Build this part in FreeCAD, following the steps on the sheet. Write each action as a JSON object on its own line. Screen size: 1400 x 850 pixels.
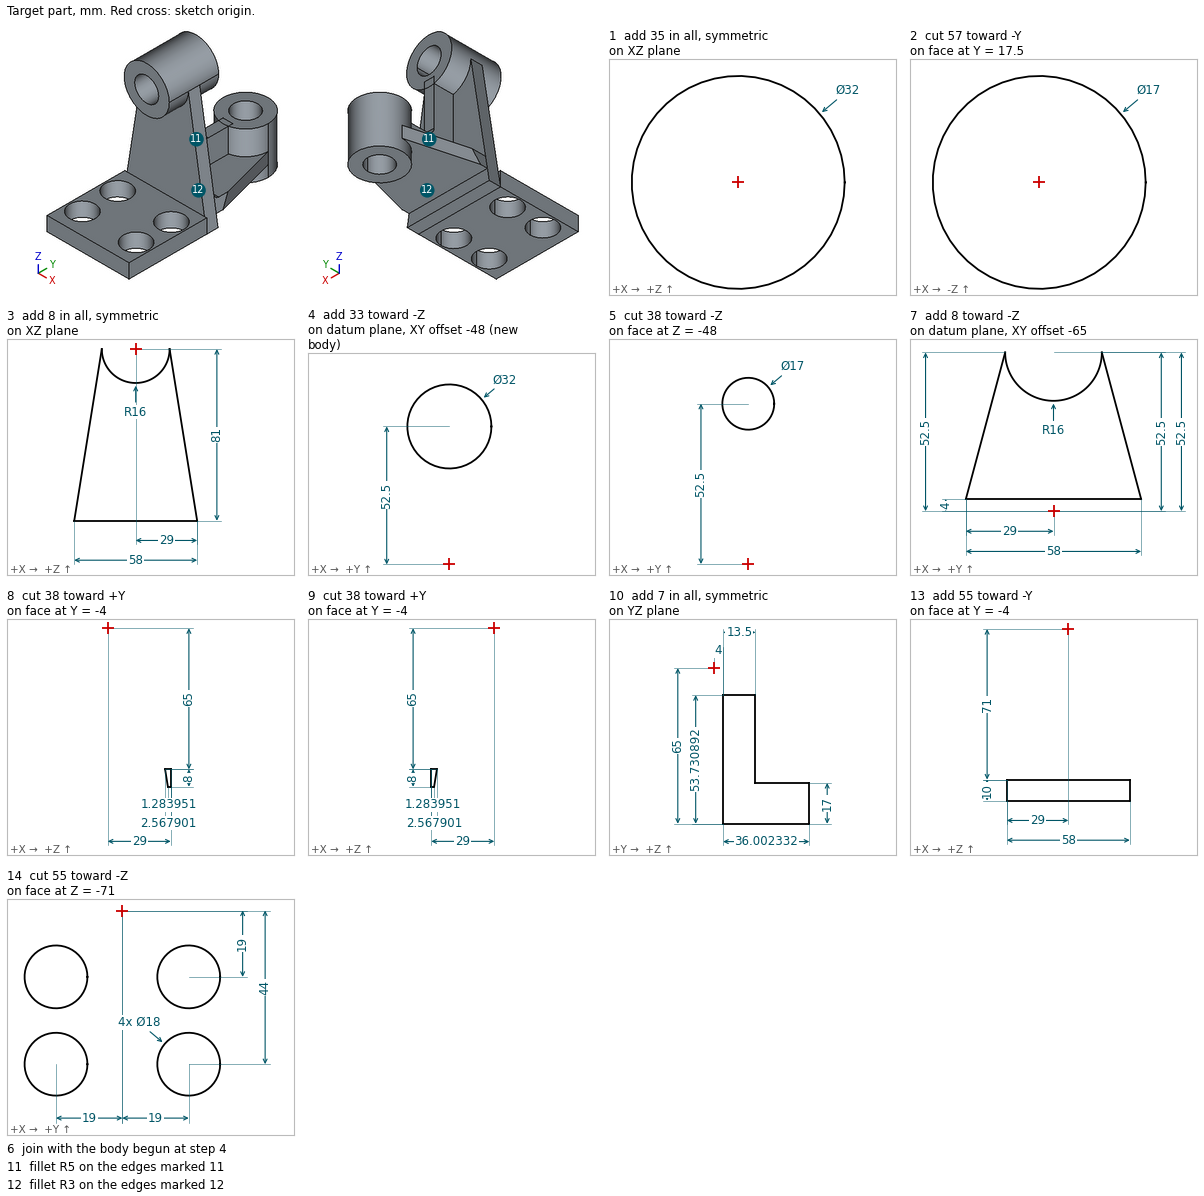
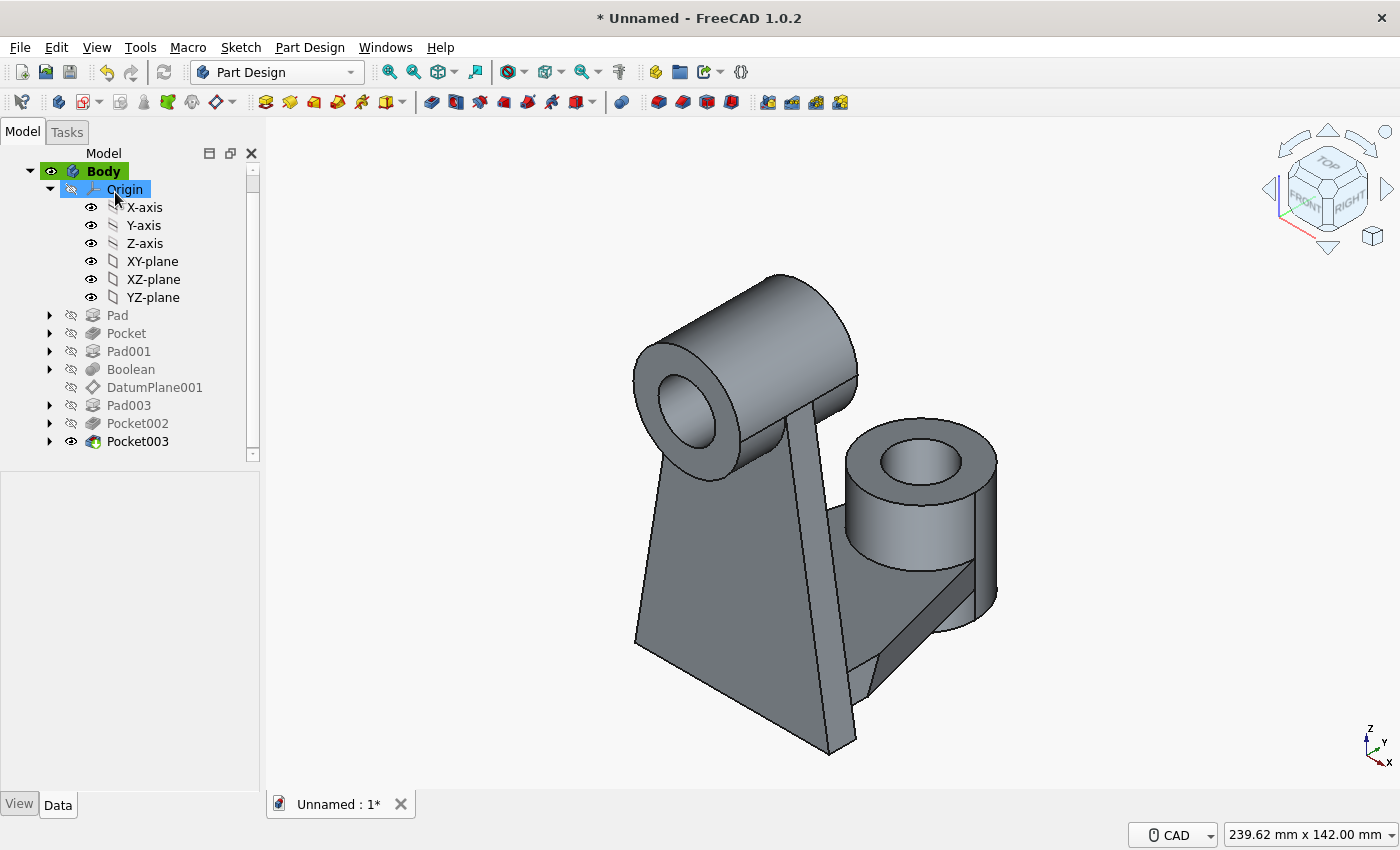
{"action": "left_click", "coordinate": [84, 102]}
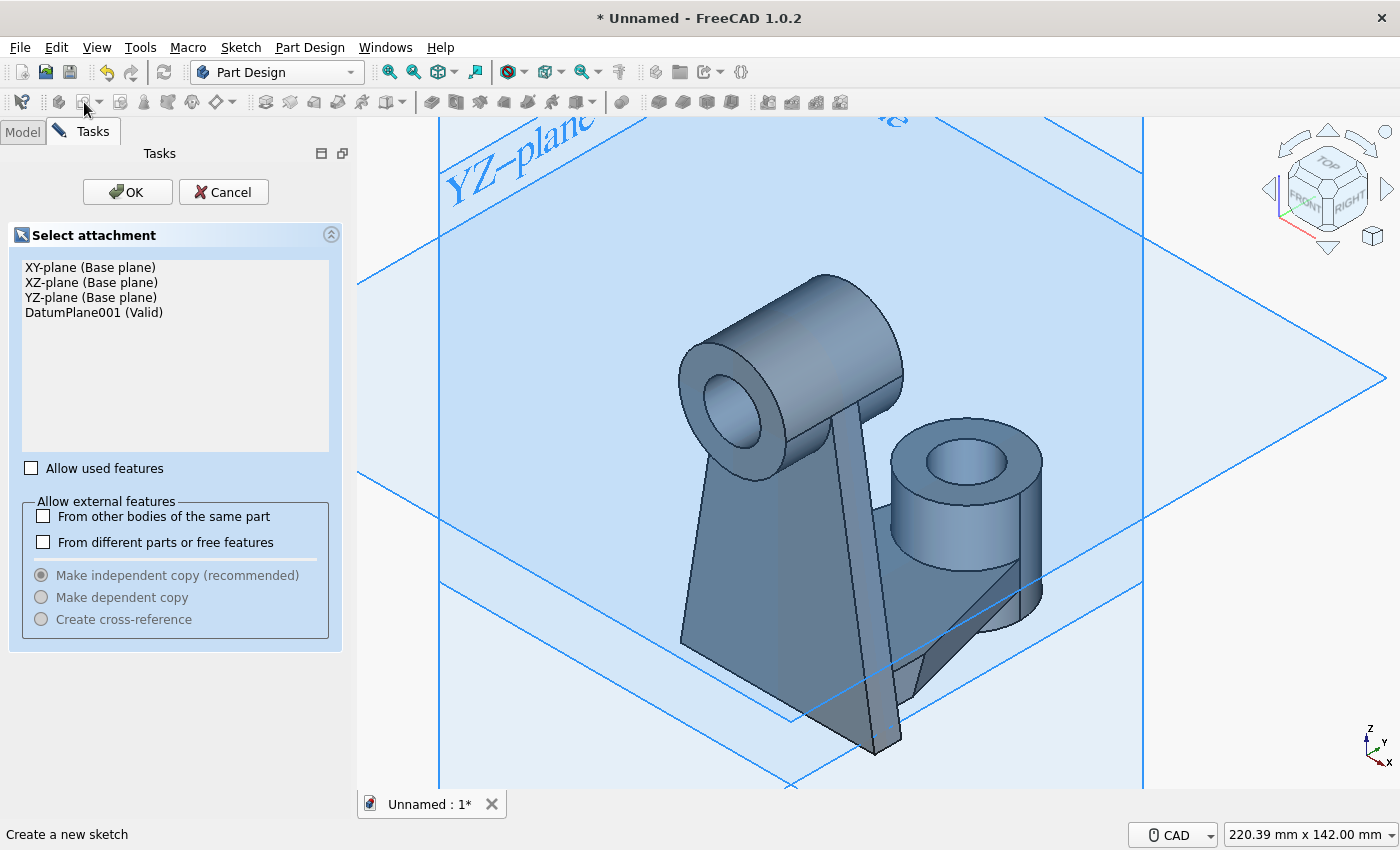
{"action": "left_click", "coordinate": [82, 298]}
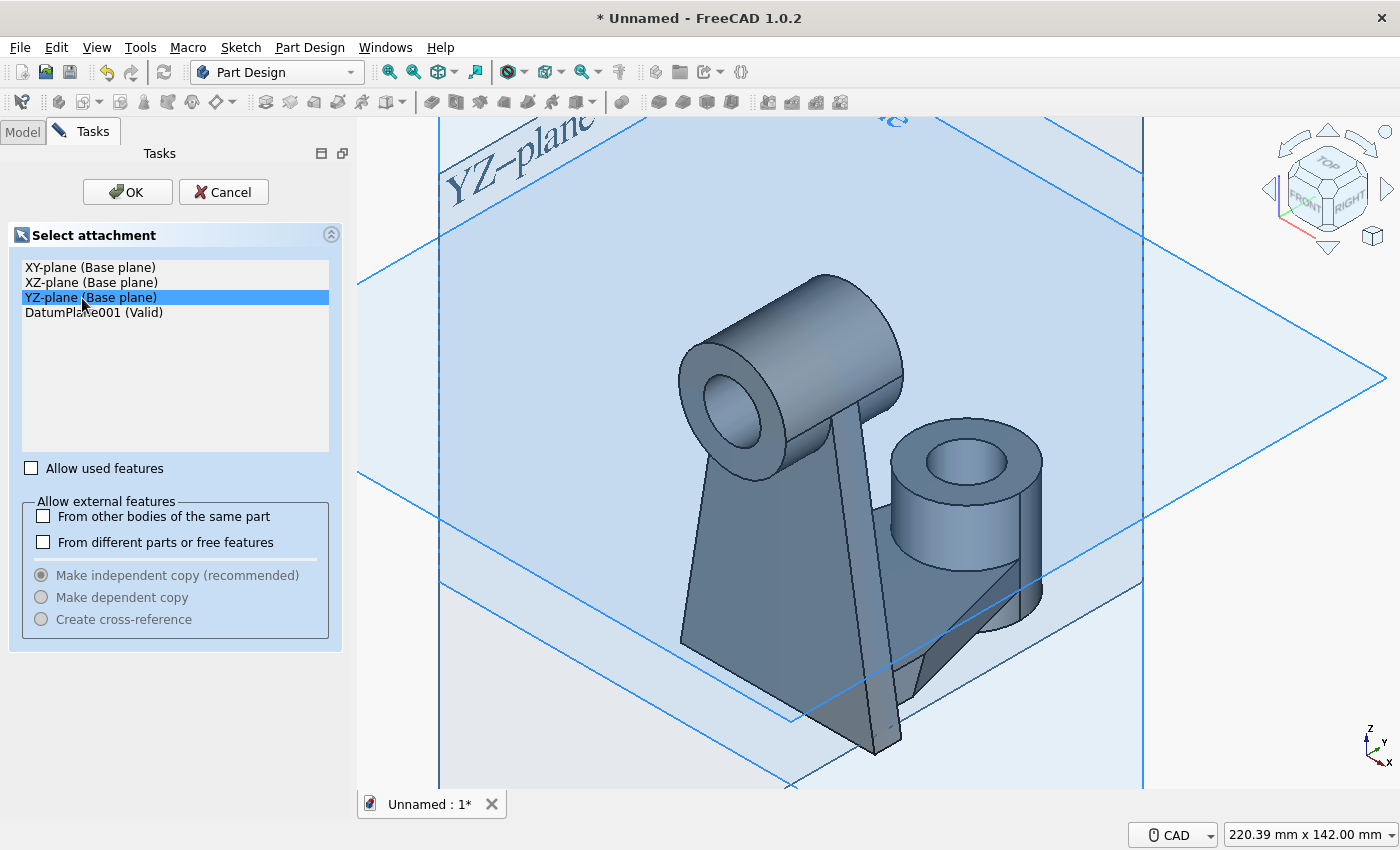
{"action": "left_click", "coordinate": [128, 192]}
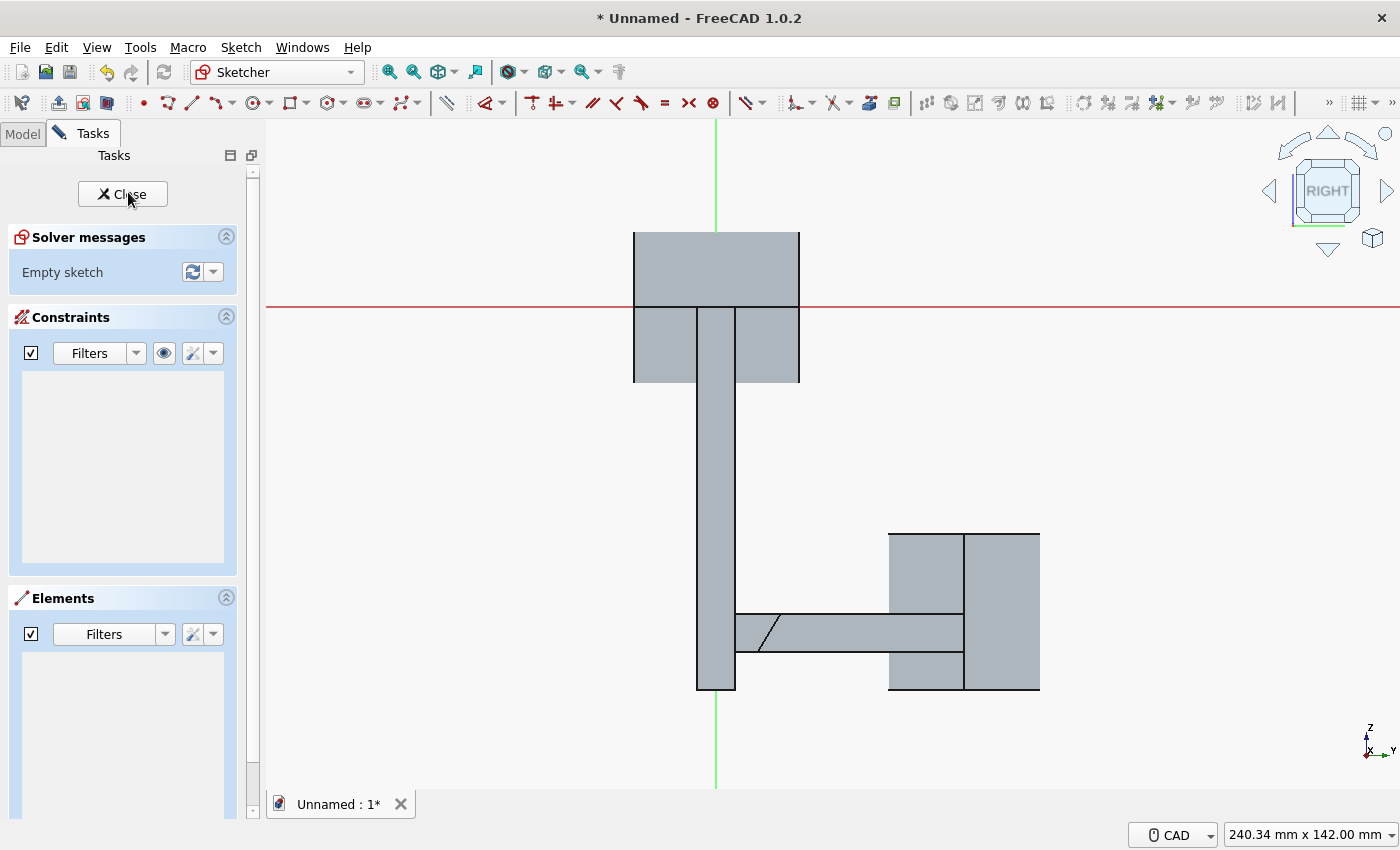
{"action": "left_click", "coordinate": [108, 104]}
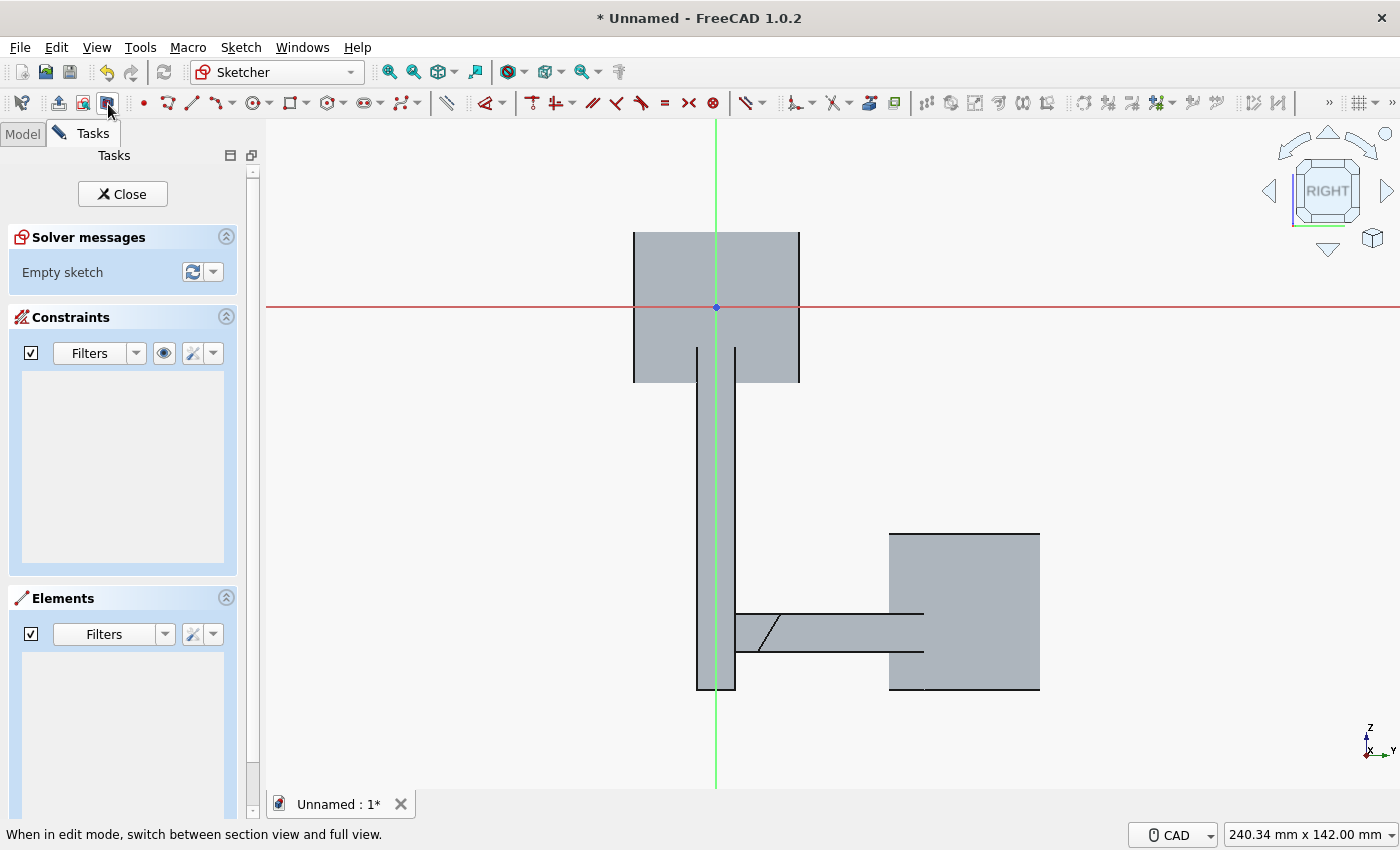
{"action": "scroll", "coordinate": [905, 474], "scroll_direction": "up", "scroll_amount": 2}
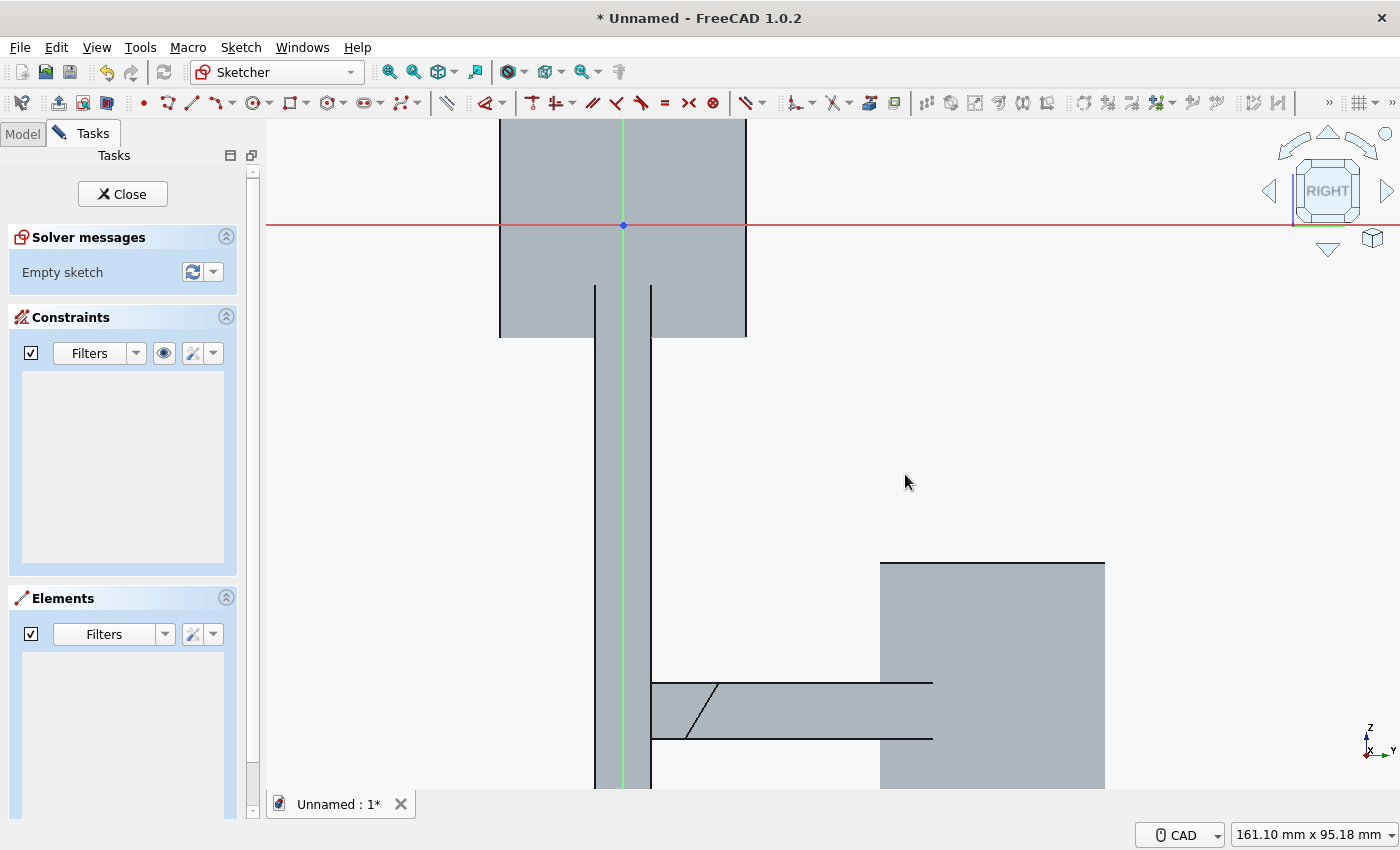
{"action": "key", "text": "g m"}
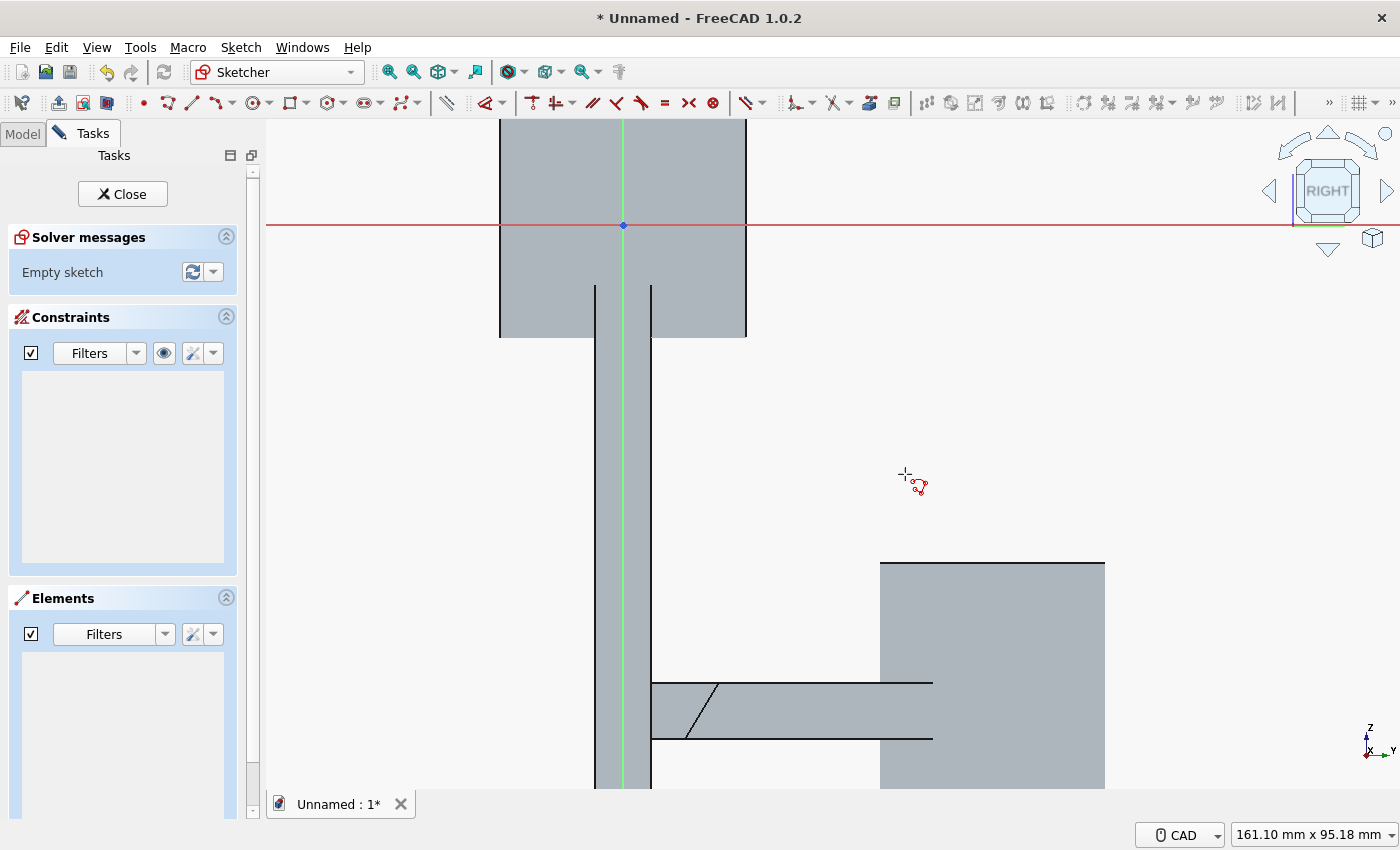
{"action": "left_click", "coordinate": [651, 304]}
{"action": "left_click", "coordinate": [651, 683]}
{"action": "left_click", "coordinate": [905, 683]}
{"action": "left_click", "coordinate": [905, 563]}
{"action": "left_click", "coordinate": [746, 563]}
{"action": "left_click", "coordinate": [746, 304]}
{"action": "left_click", "coordinate": [651, 305]}
{"action": "key", "text": "Escape"}
{"action": "key", "text": "Escape"}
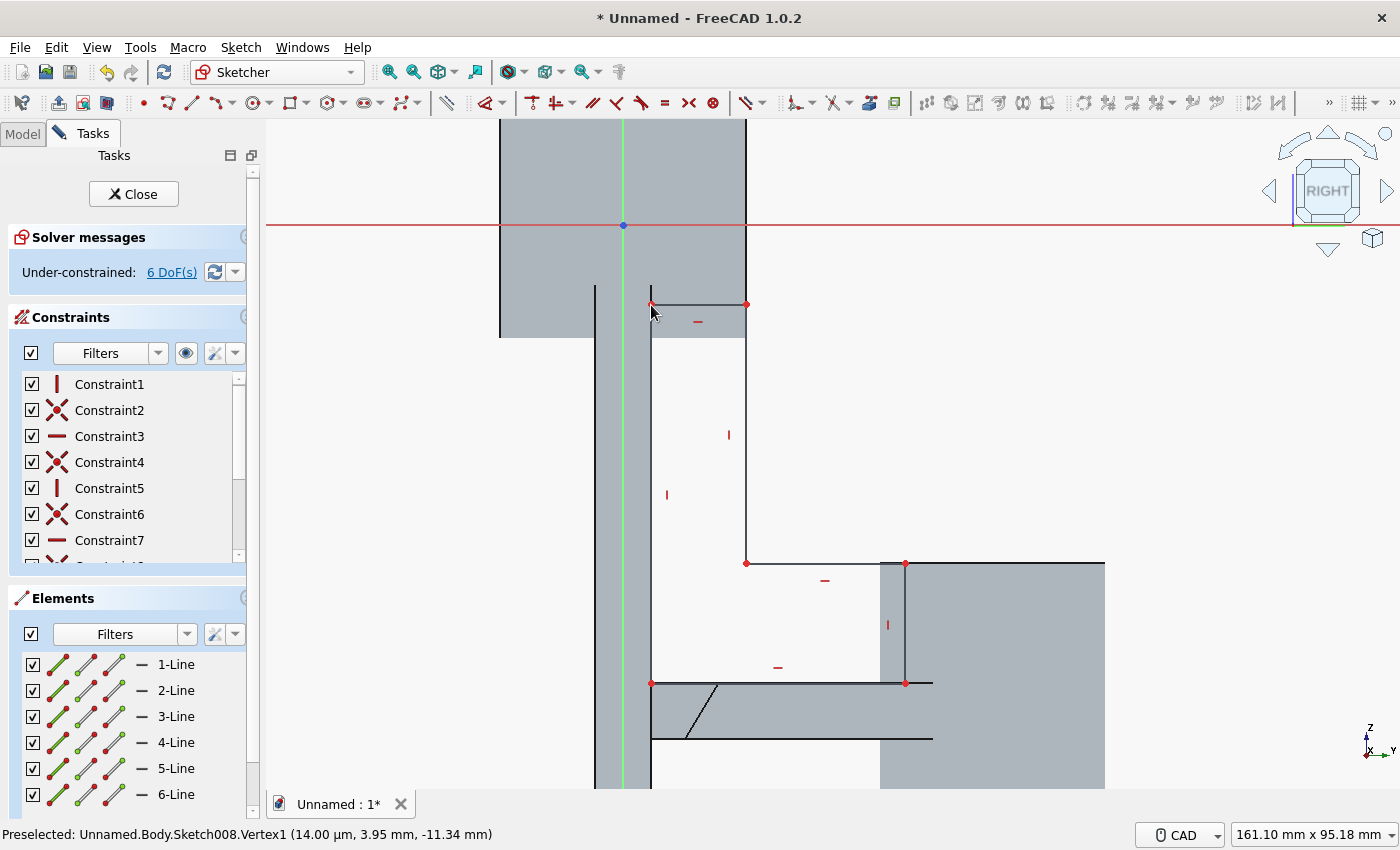
{"action": "key", "text": "d"}